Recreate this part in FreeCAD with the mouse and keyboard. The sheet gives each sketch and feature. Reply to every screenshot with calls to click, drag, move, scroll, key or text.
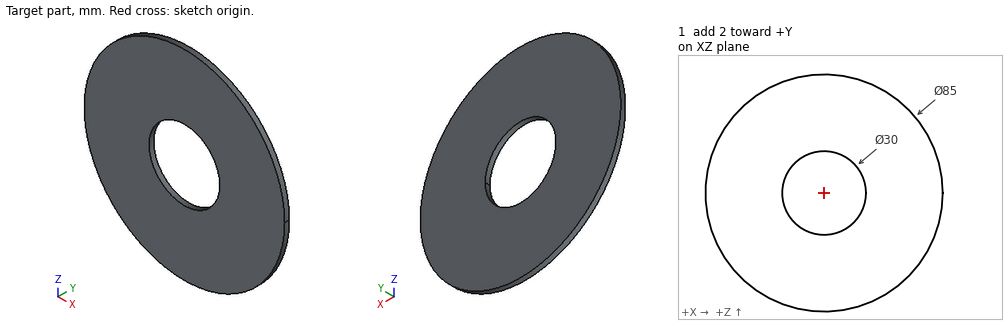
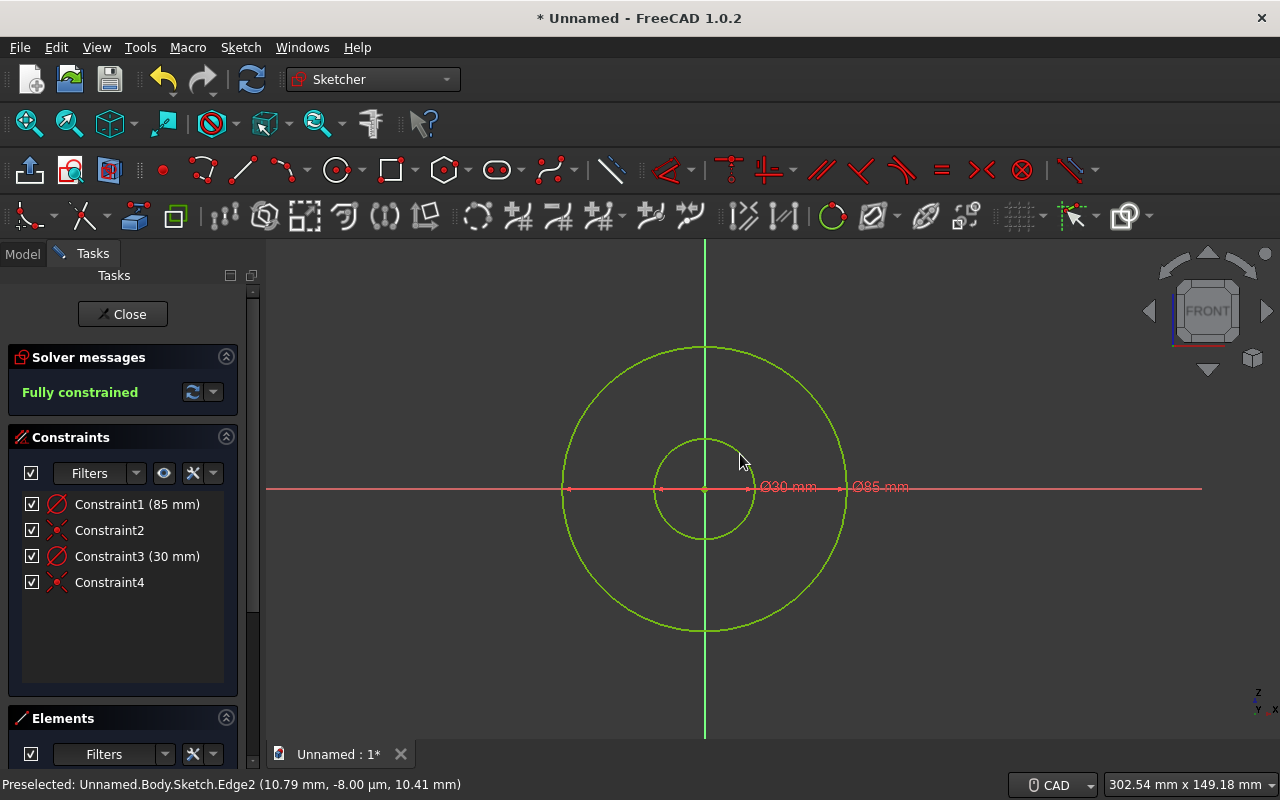
click(123, 314)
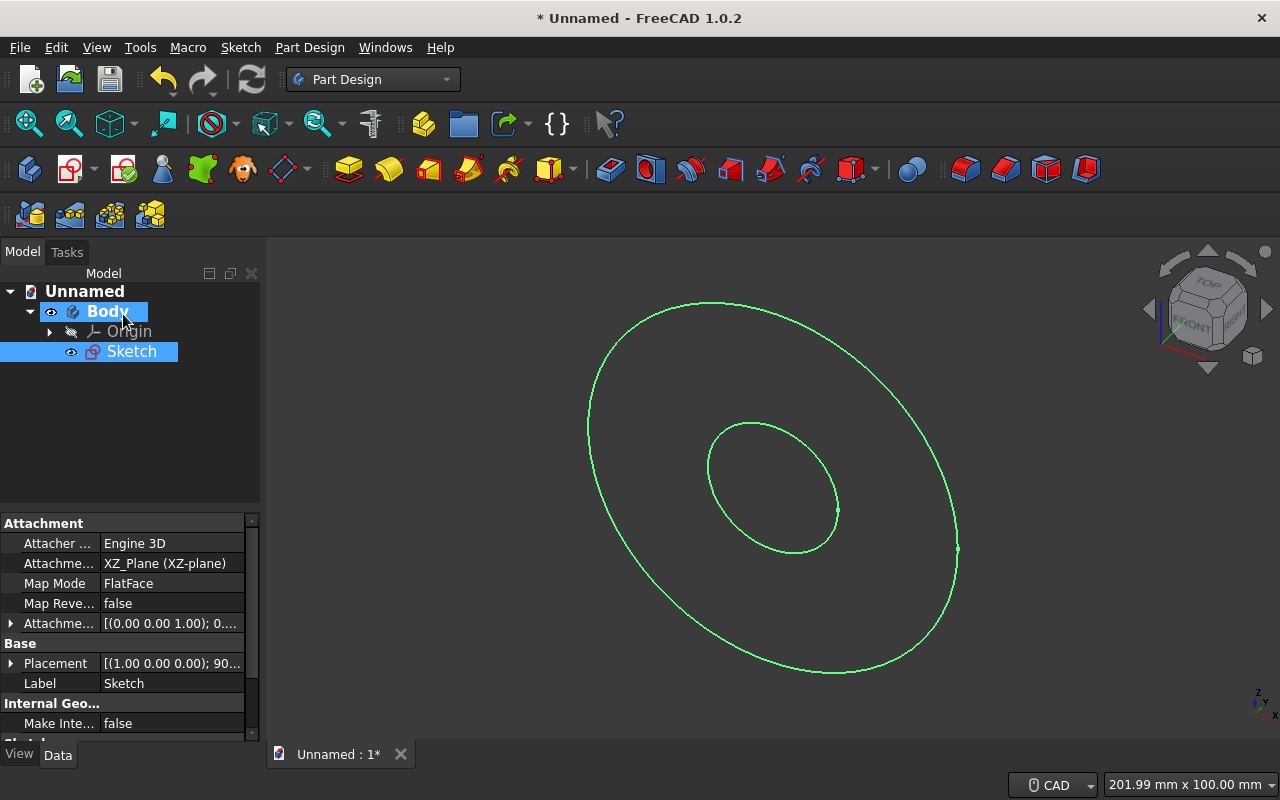
click(350, 170)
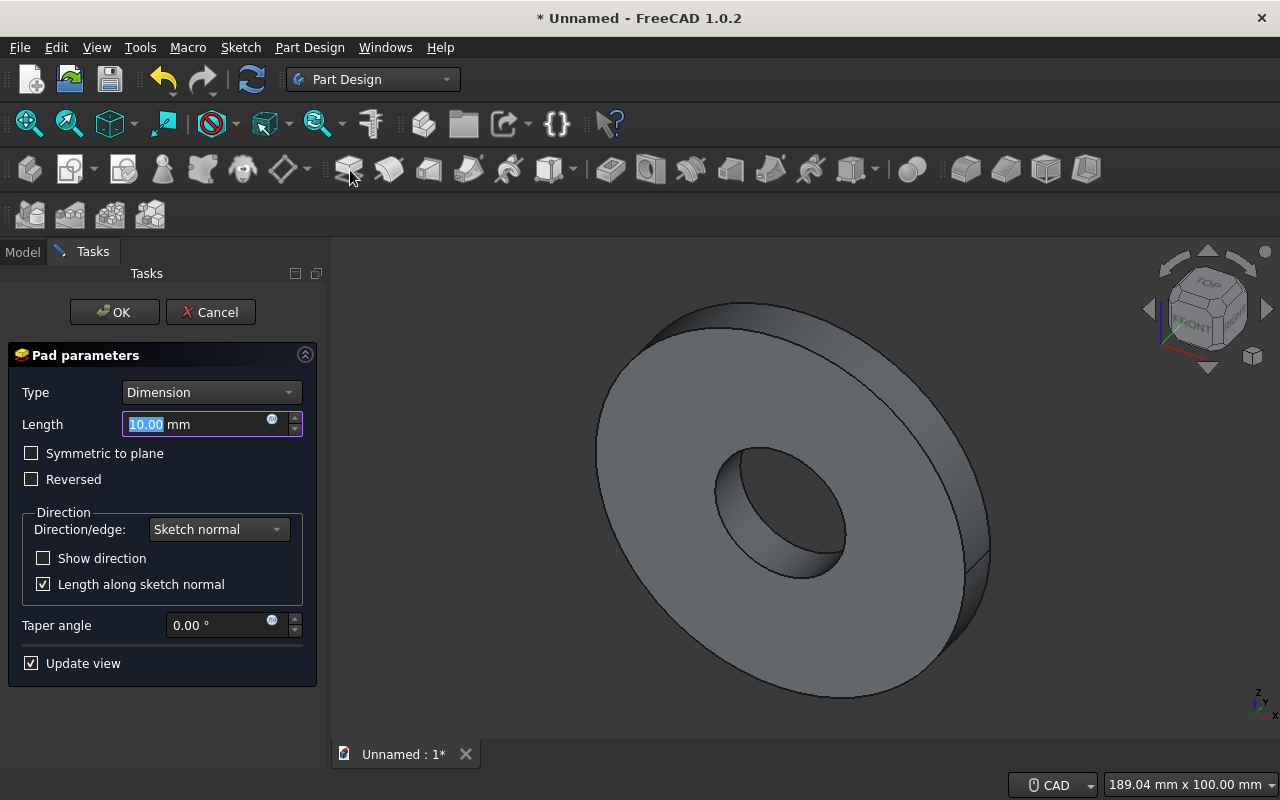
text(2)
key(Tab)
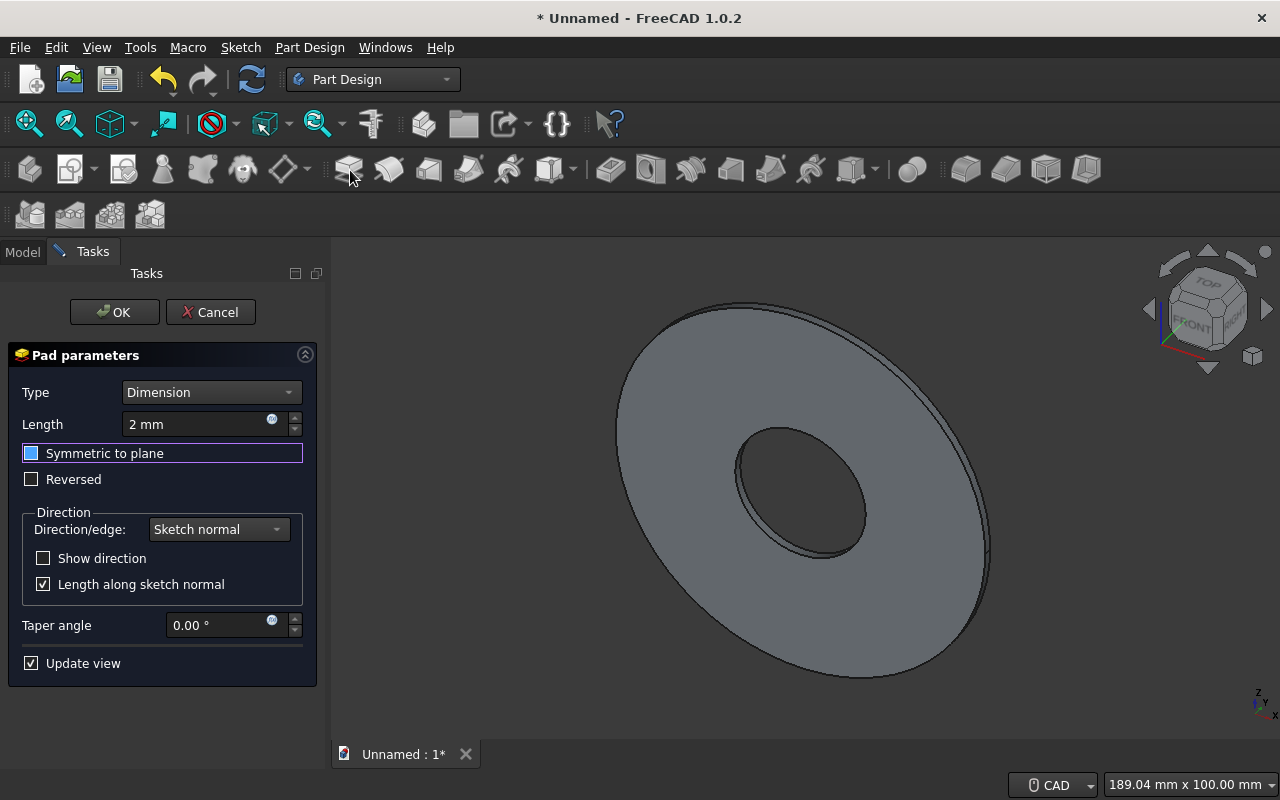
click(30, 479)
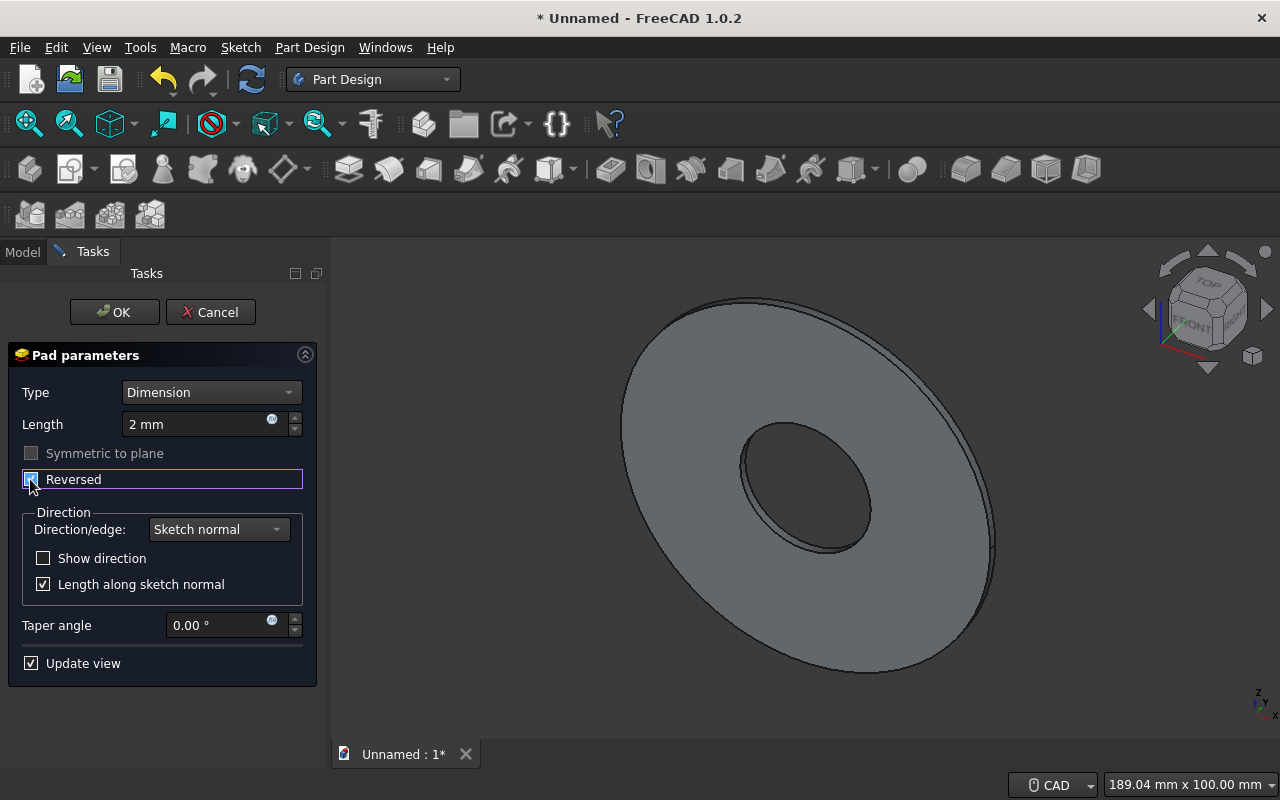
click(115, 312)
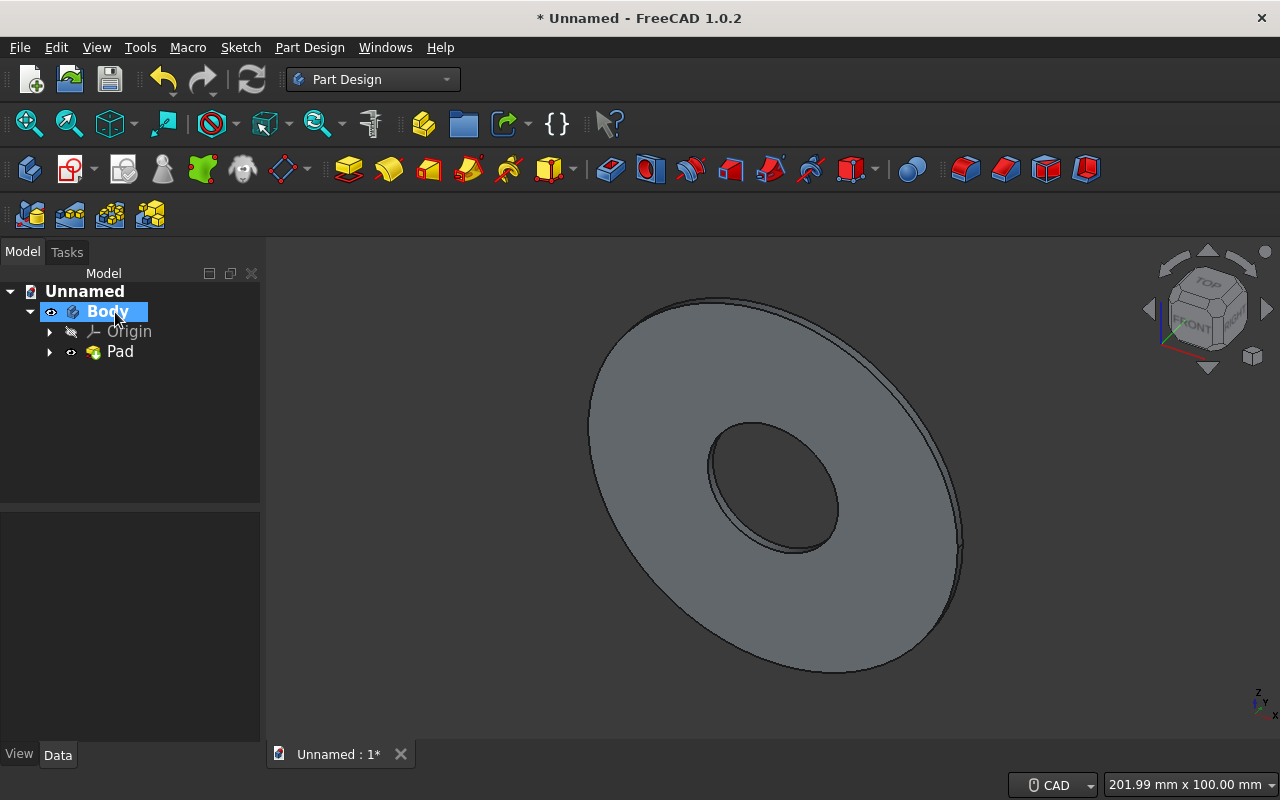
key(0)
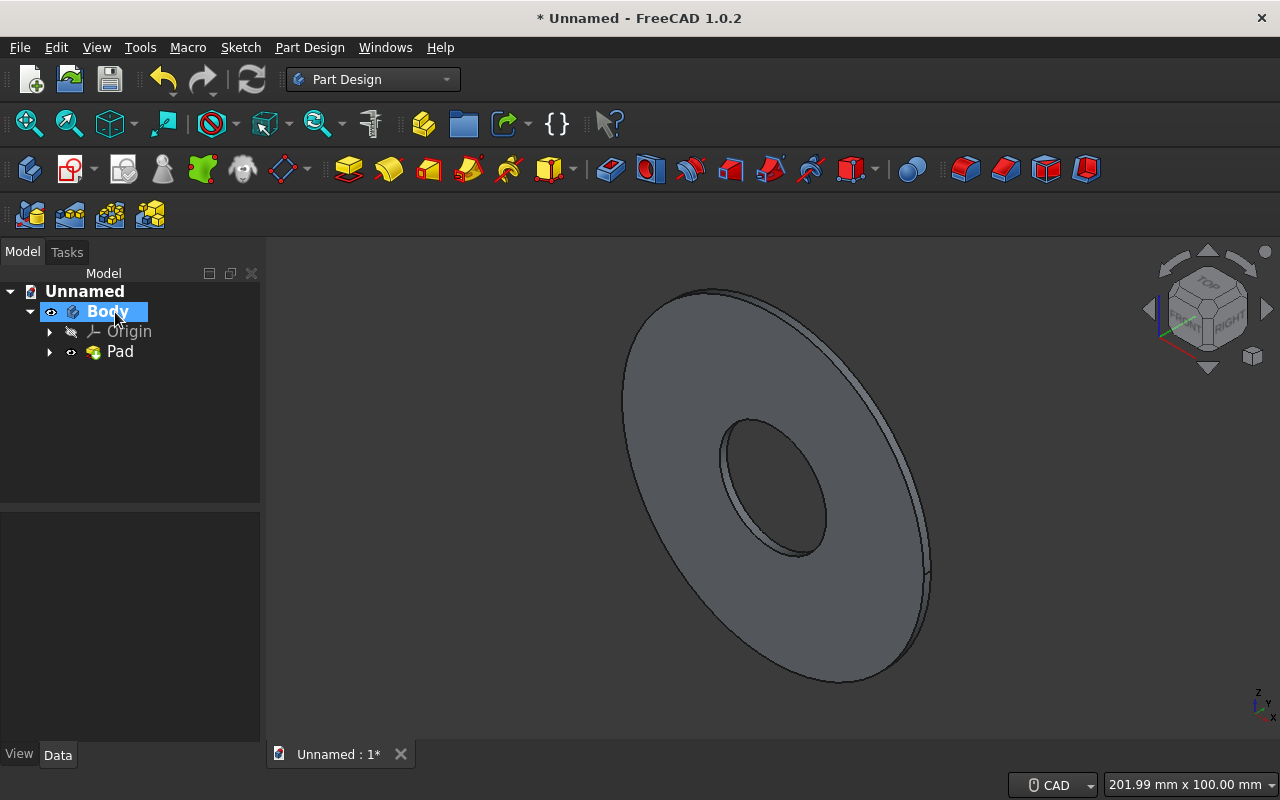
click(30, 124)